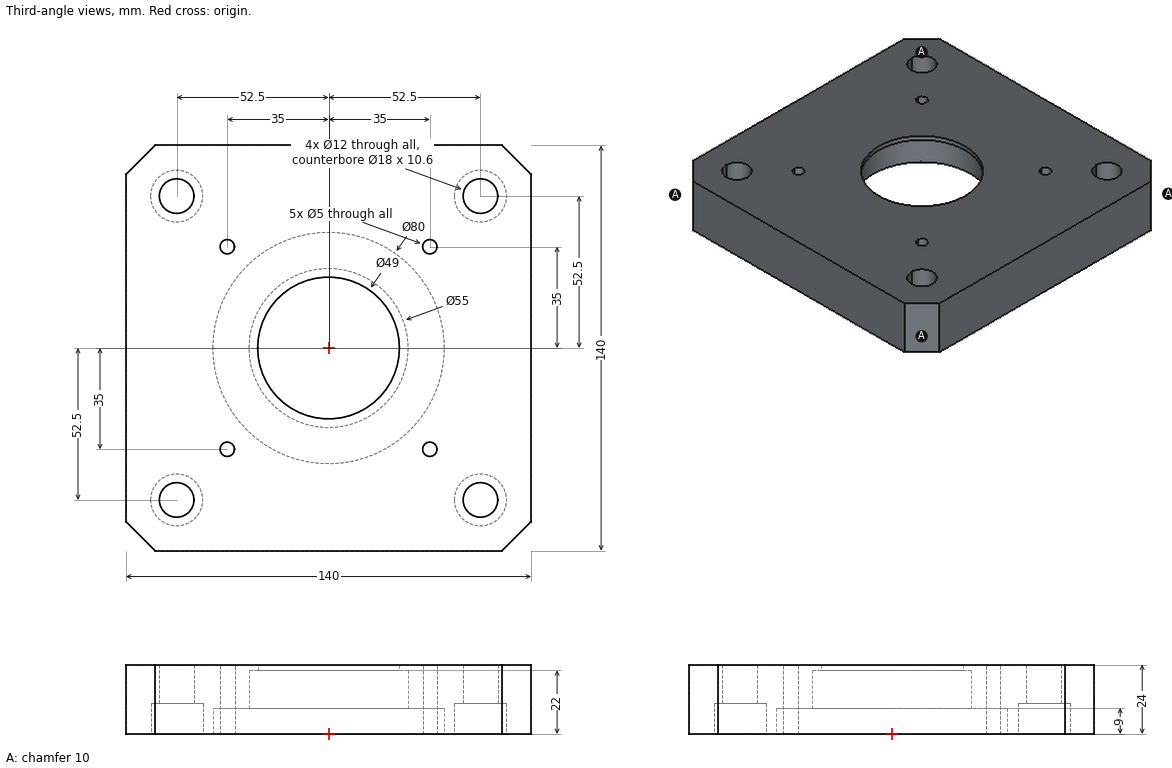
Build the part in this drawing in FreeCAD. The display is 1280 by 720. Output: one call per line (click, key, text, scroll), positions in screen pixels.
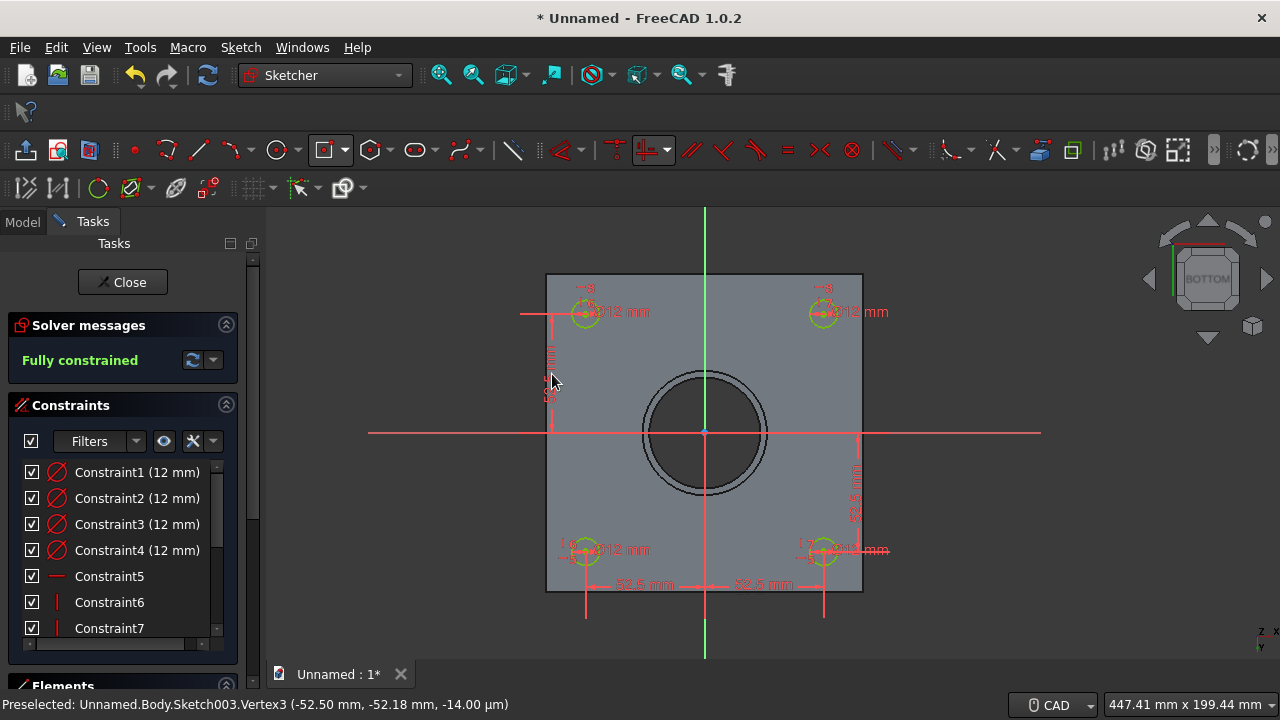
click(123, 282)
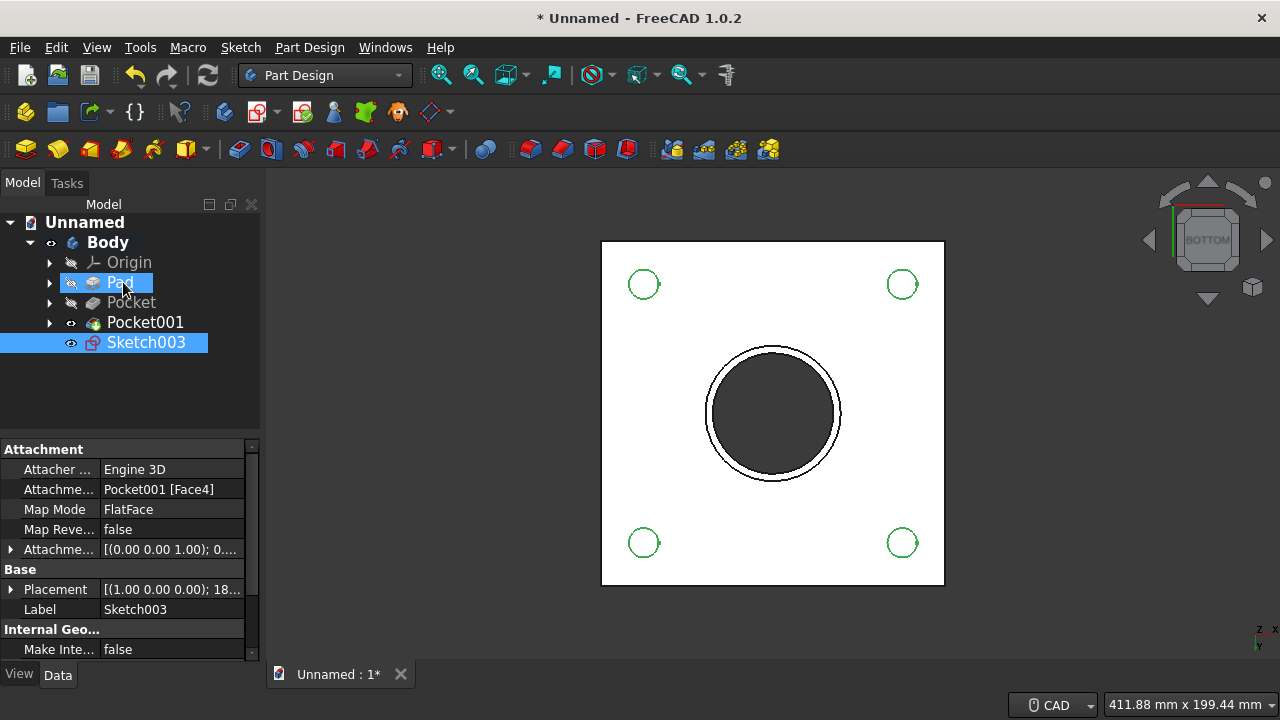
click(272, 150)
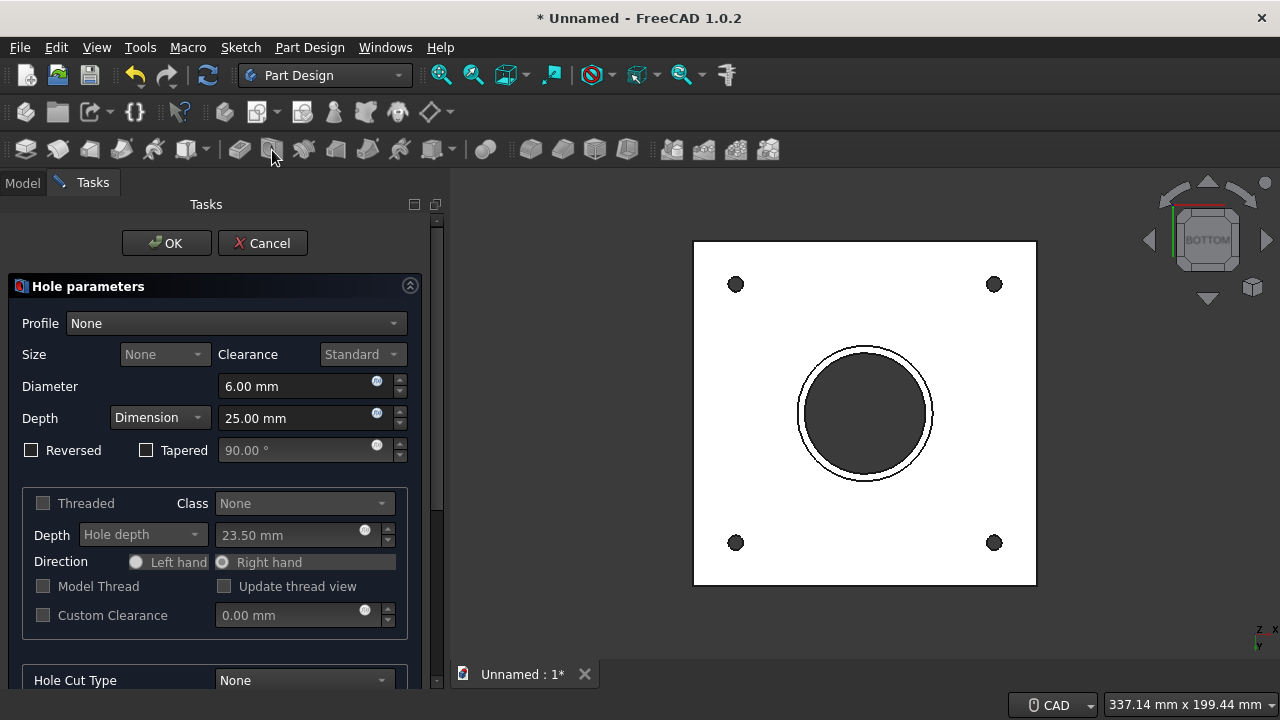
triple_click(305, 386)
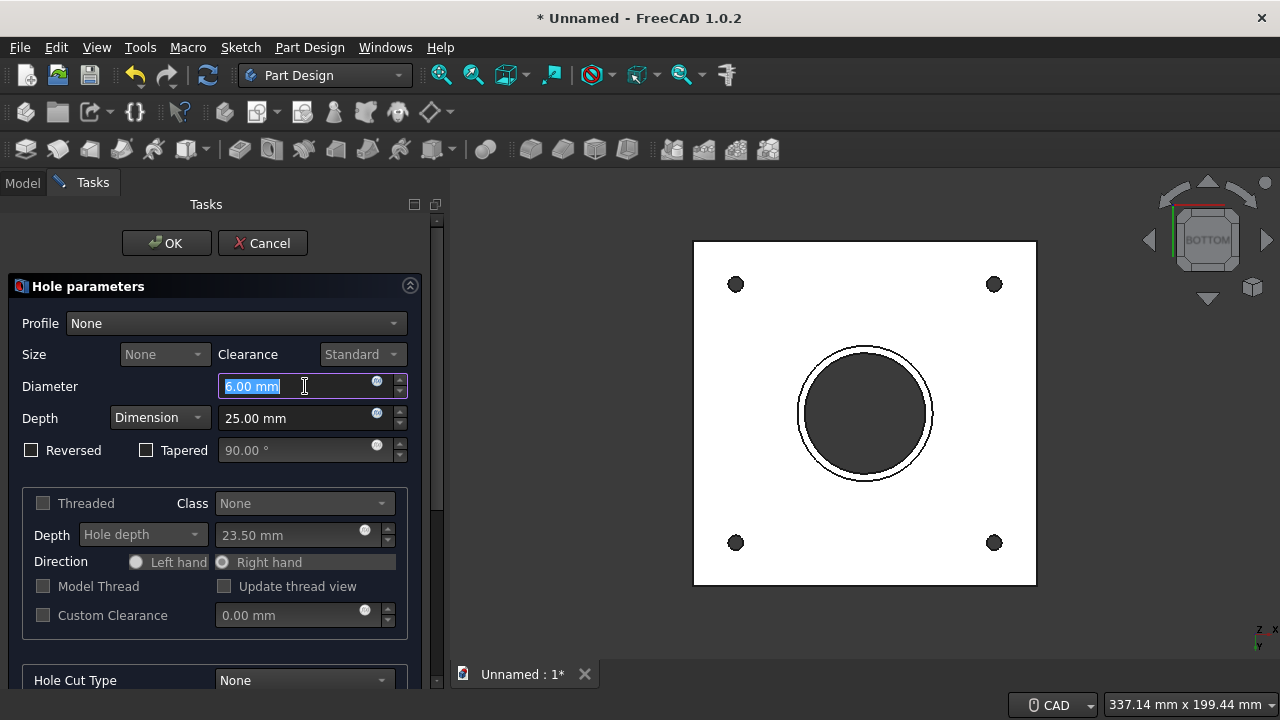
text(12)
key(Tab)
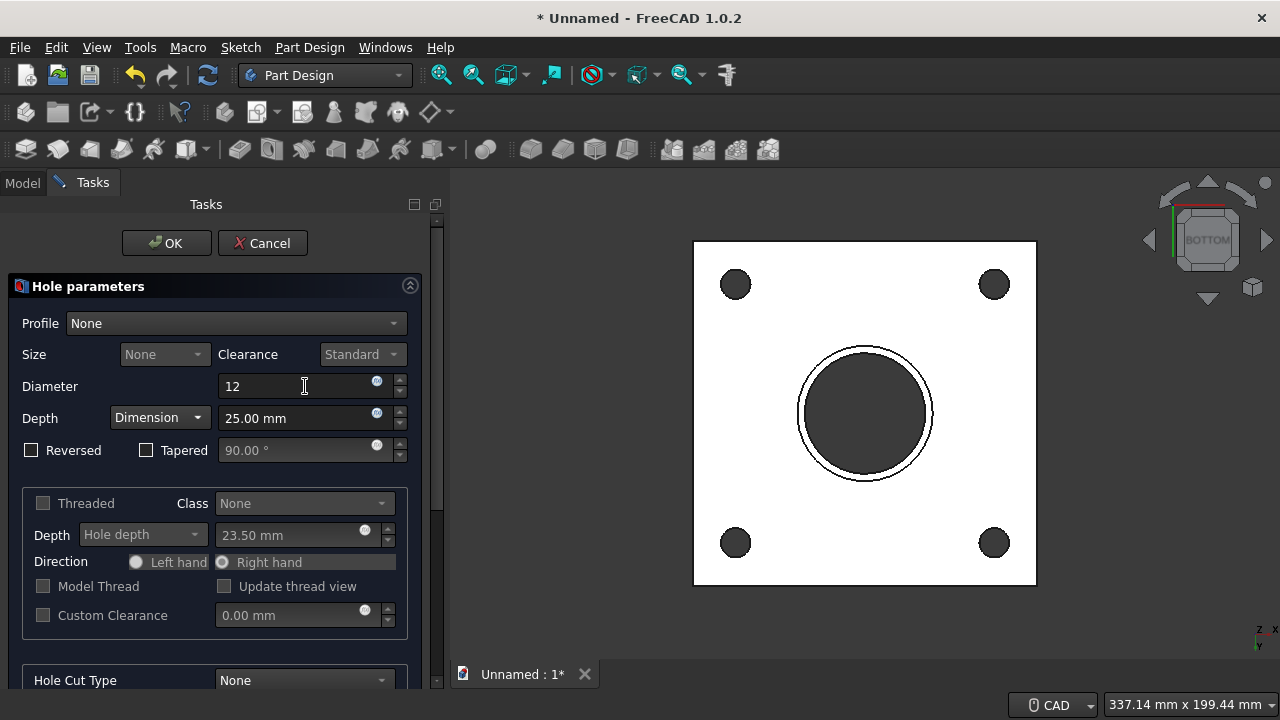
click(161, 418)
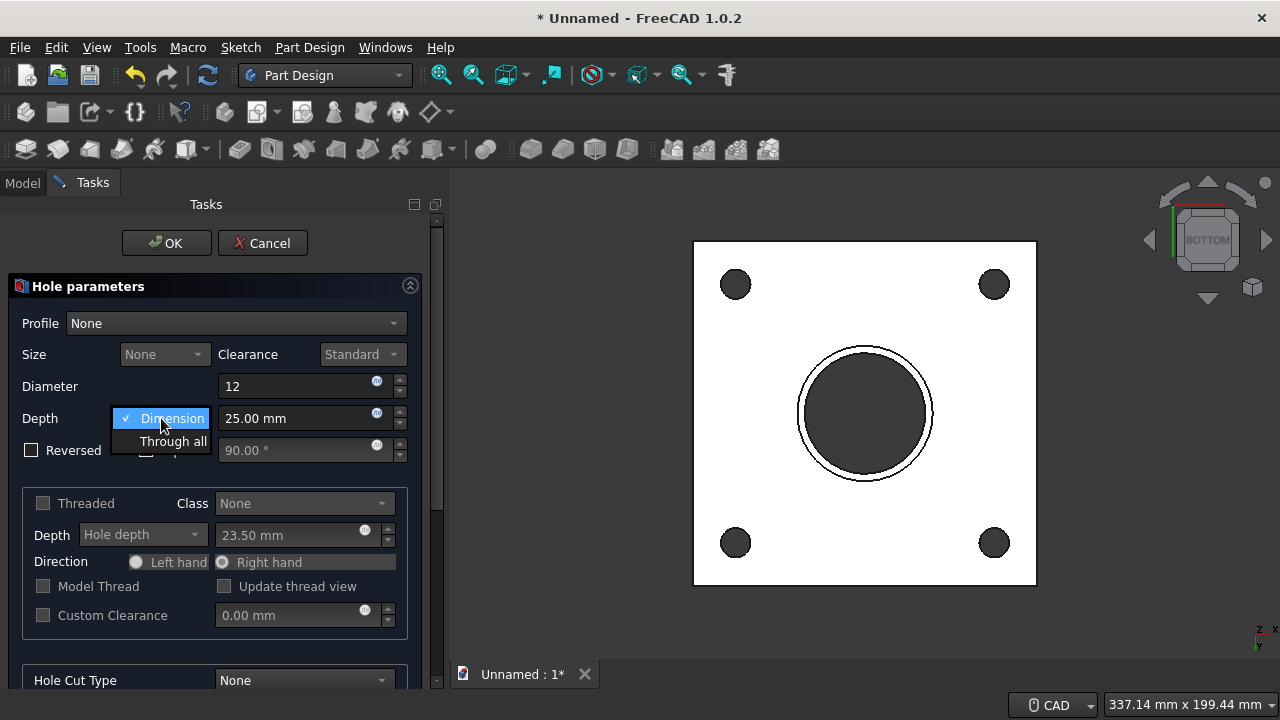
click(160, 442)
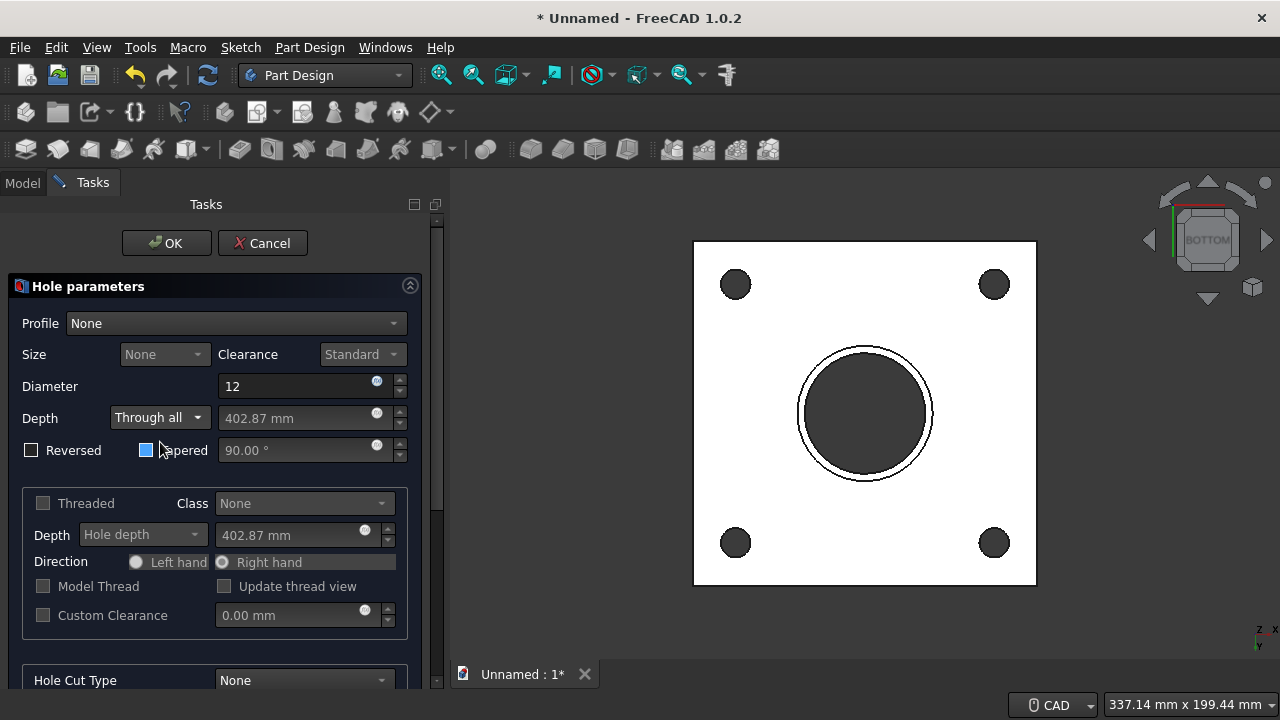
scroll(437, 451, down, 2)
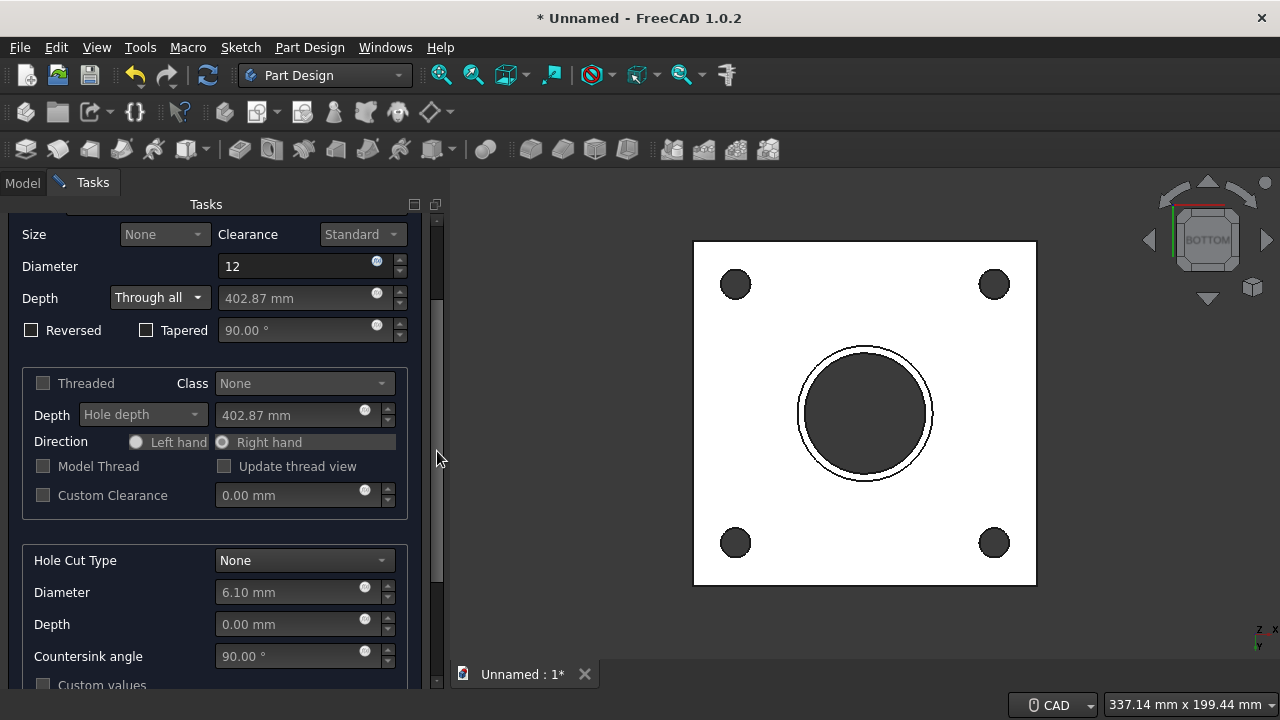
click(306, 560)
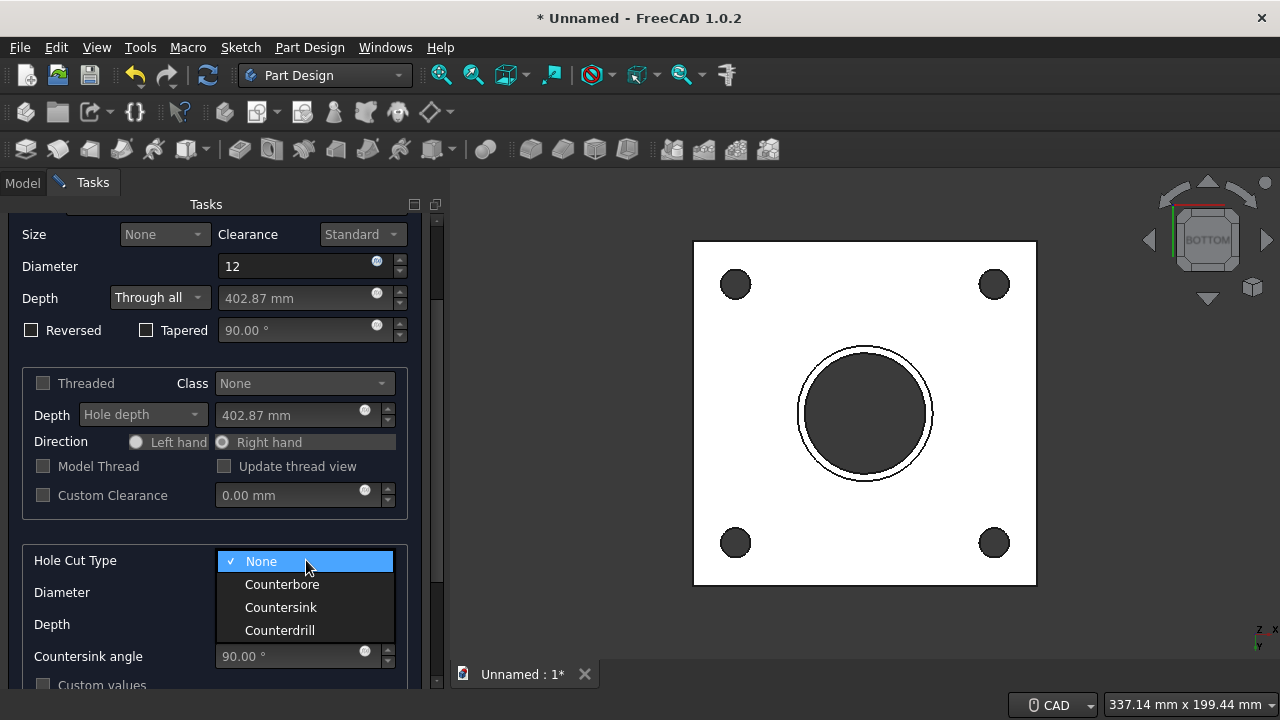
click(304, 584)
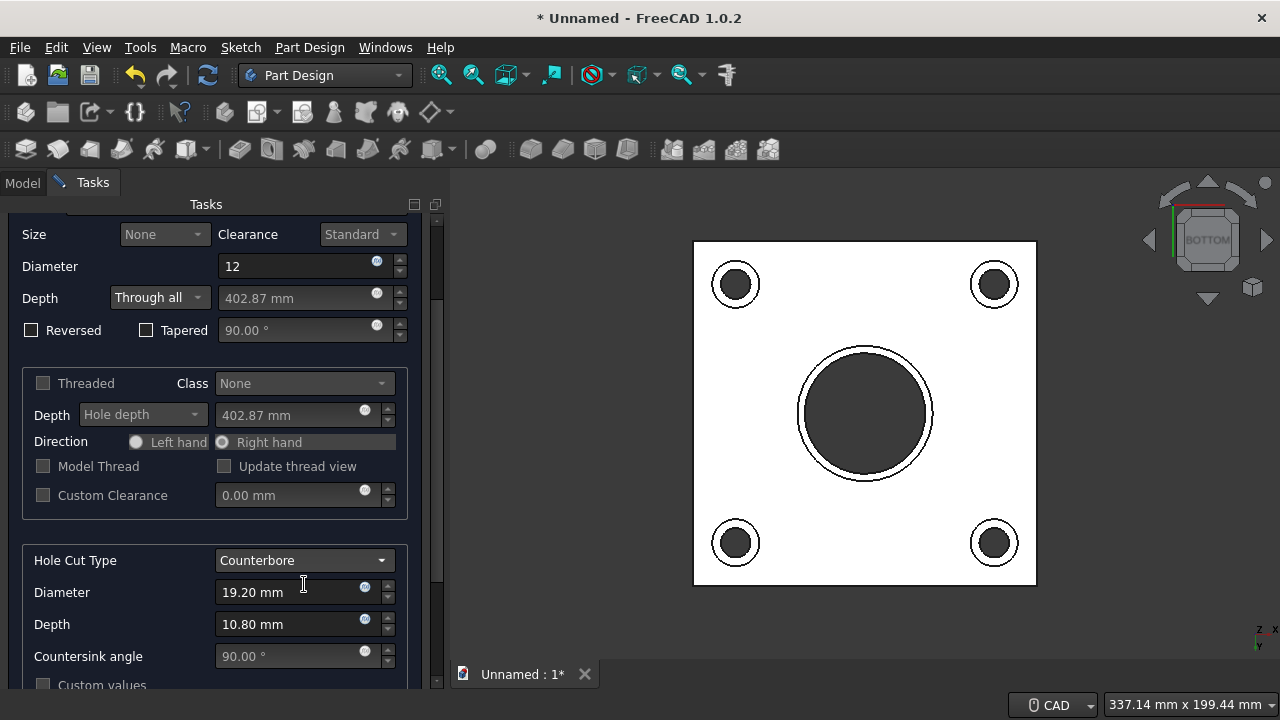
triple_click(298, 592)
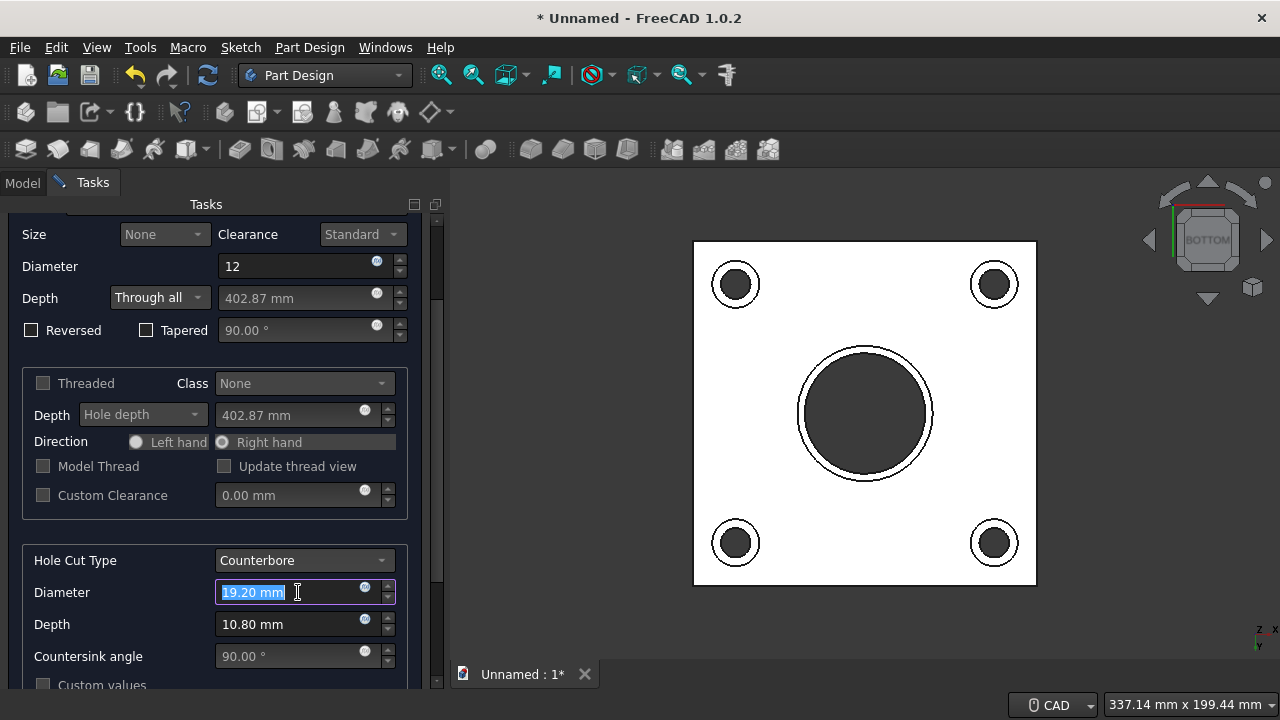
text(18)
key(Tab)